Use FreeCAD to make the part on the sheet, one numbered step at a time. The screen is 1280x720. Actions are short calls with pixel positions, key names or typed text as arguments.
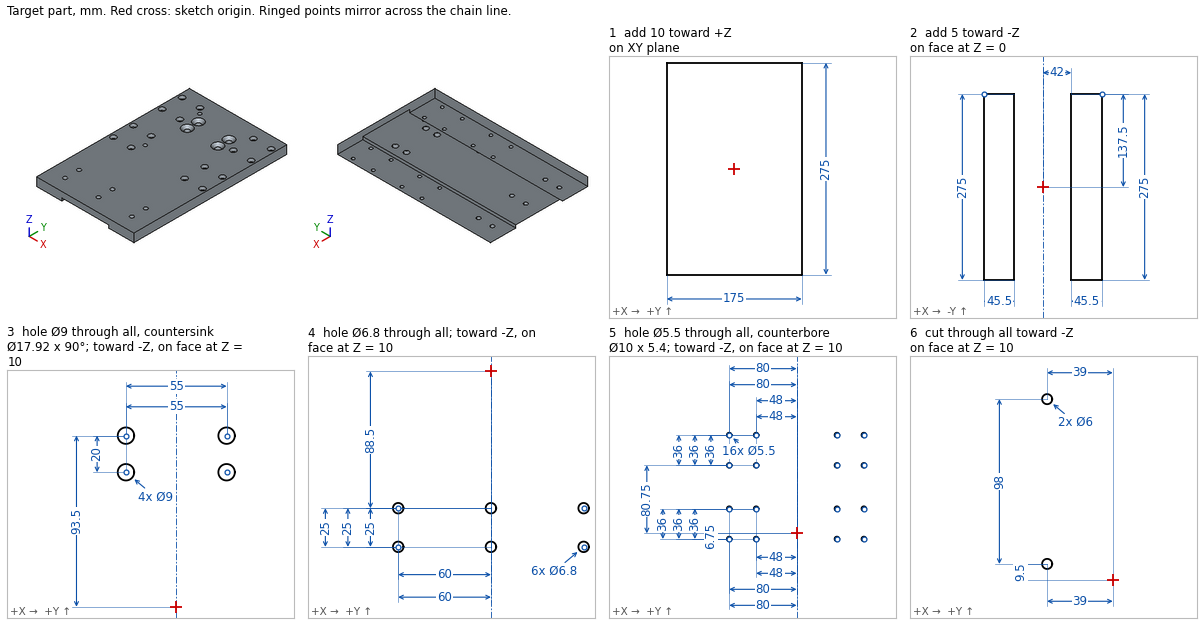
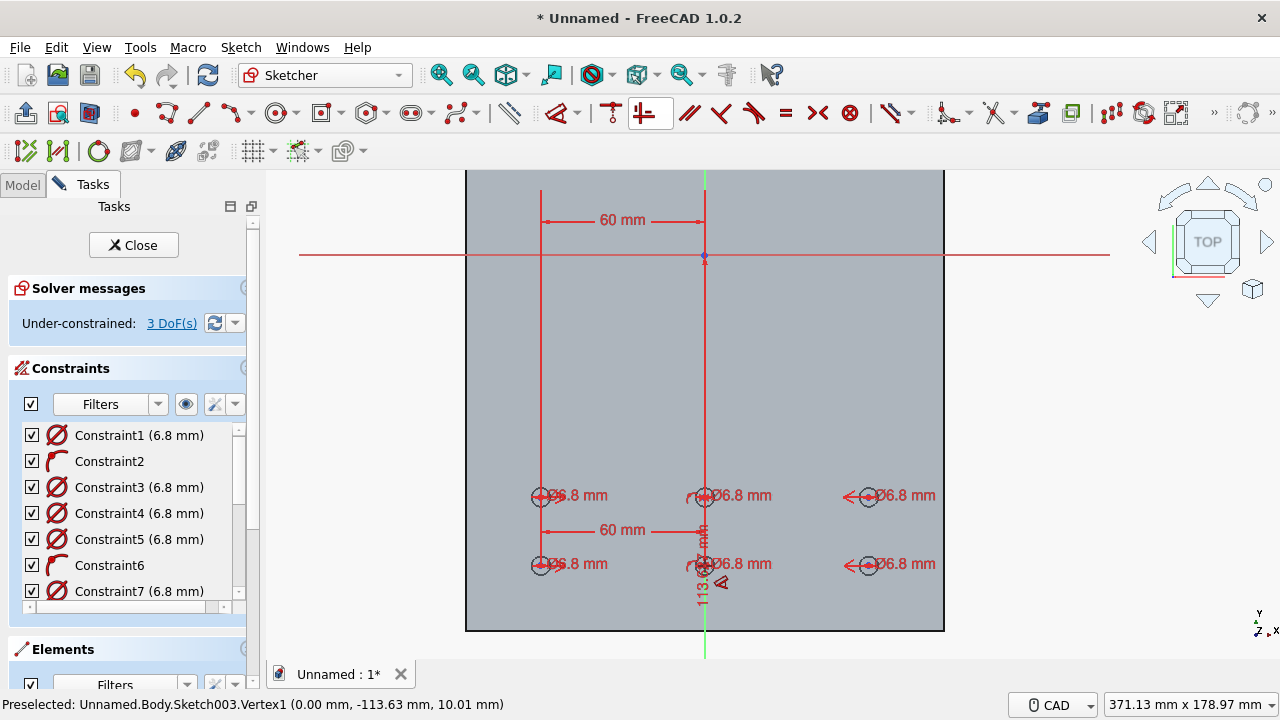
click(705, 497)
click(739, 532)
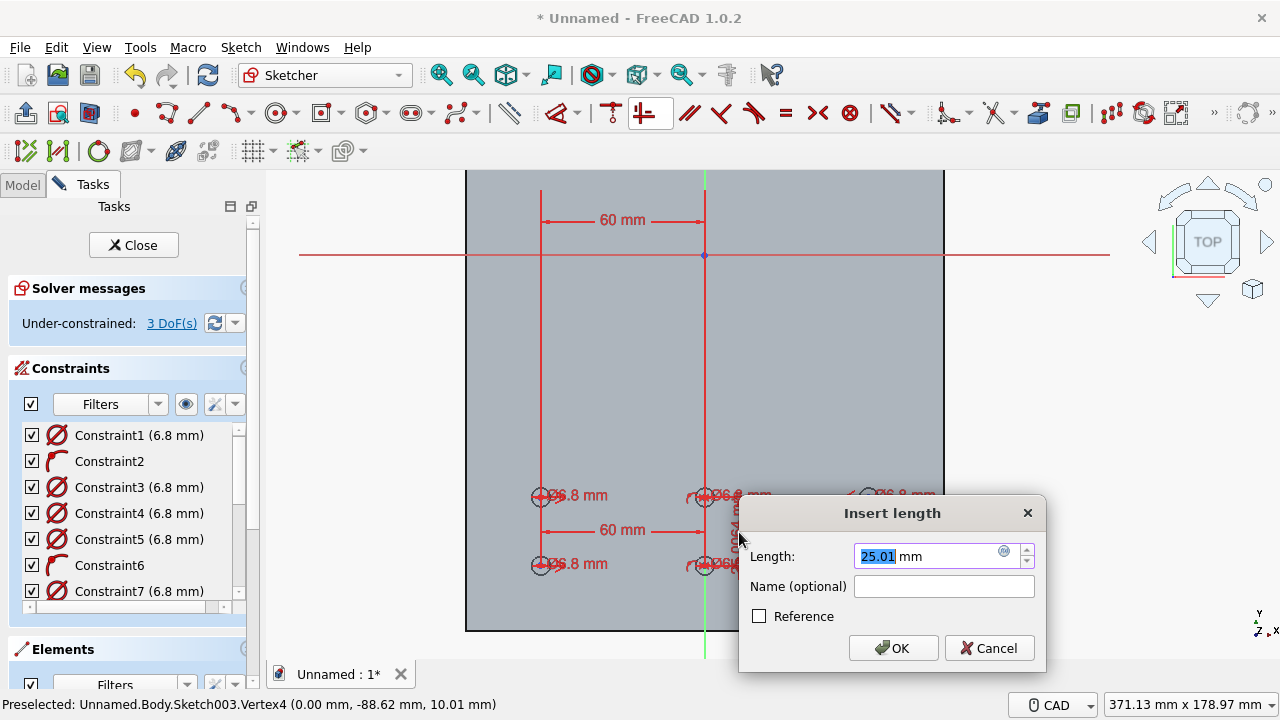
text(25)
key(Return)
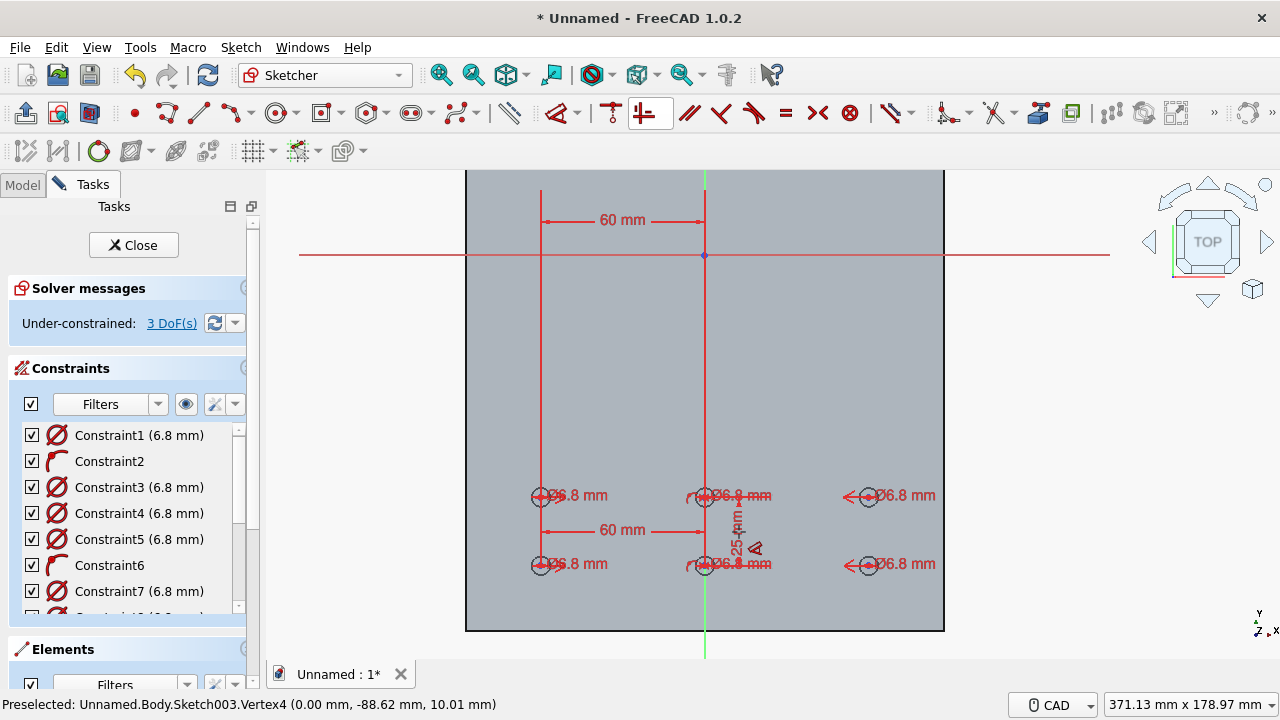
click(541, 566)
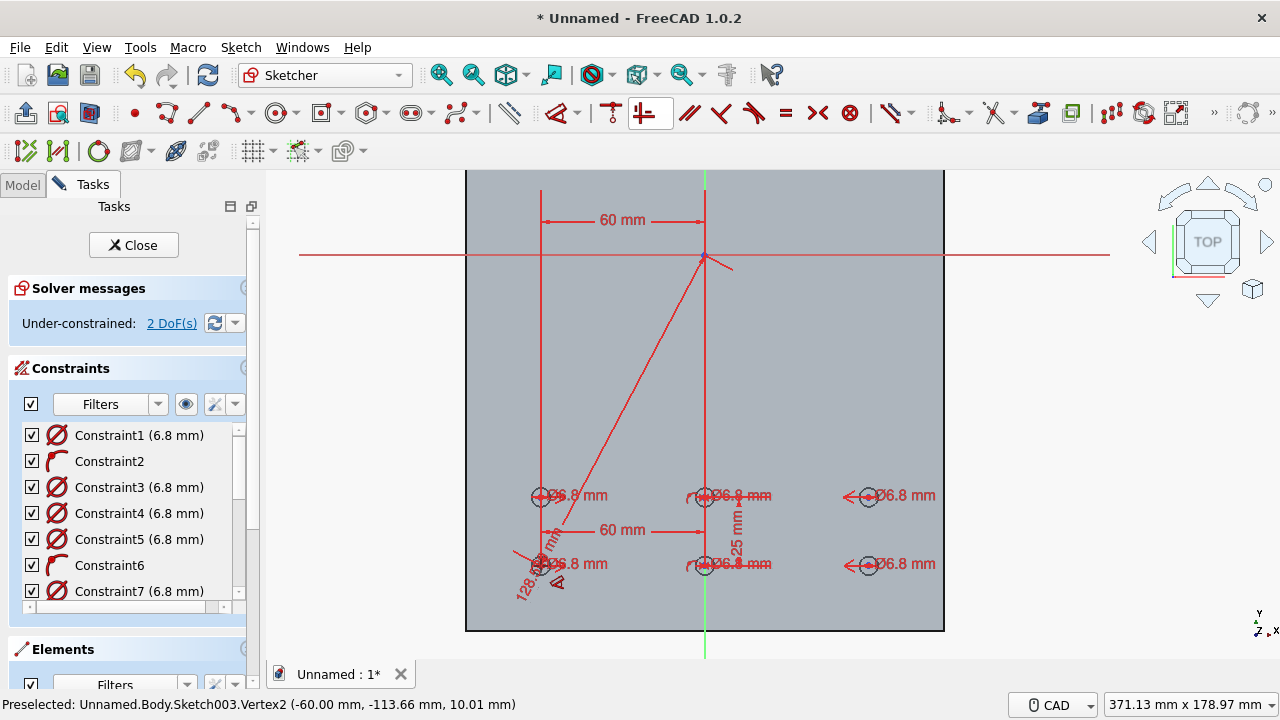
click(705, 497)
click(507, 532)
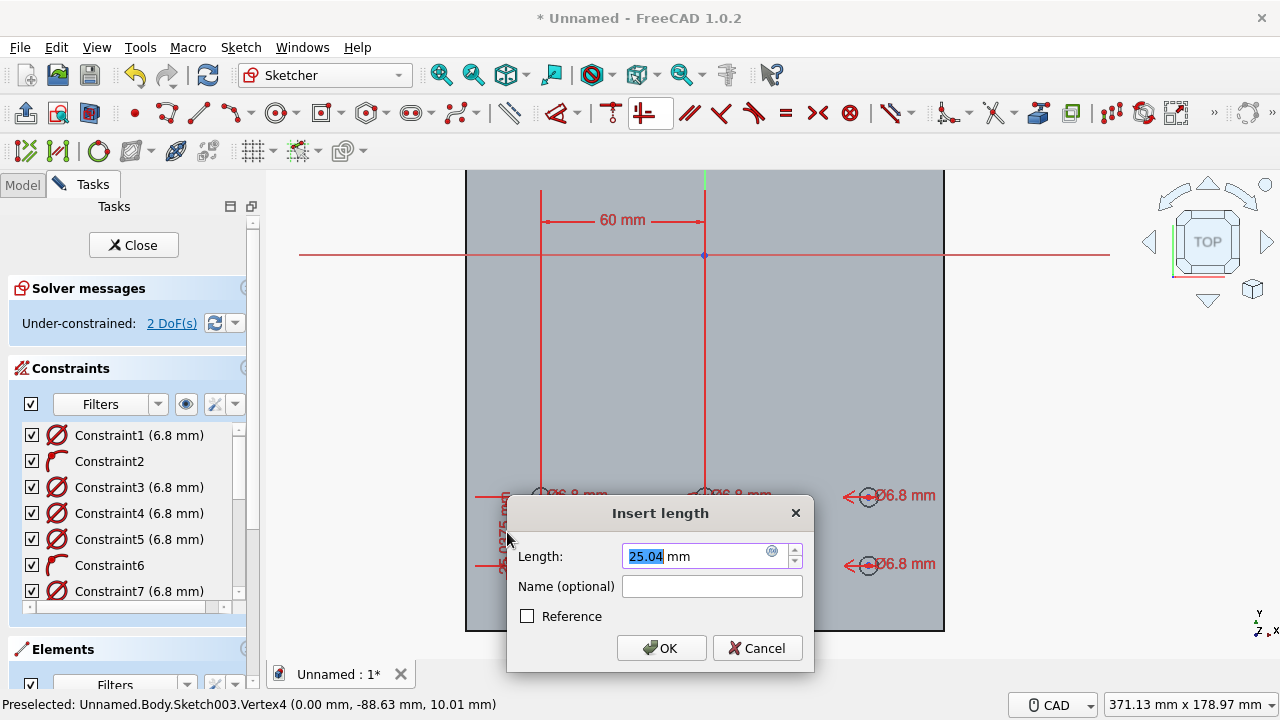
text(25)
key(Return)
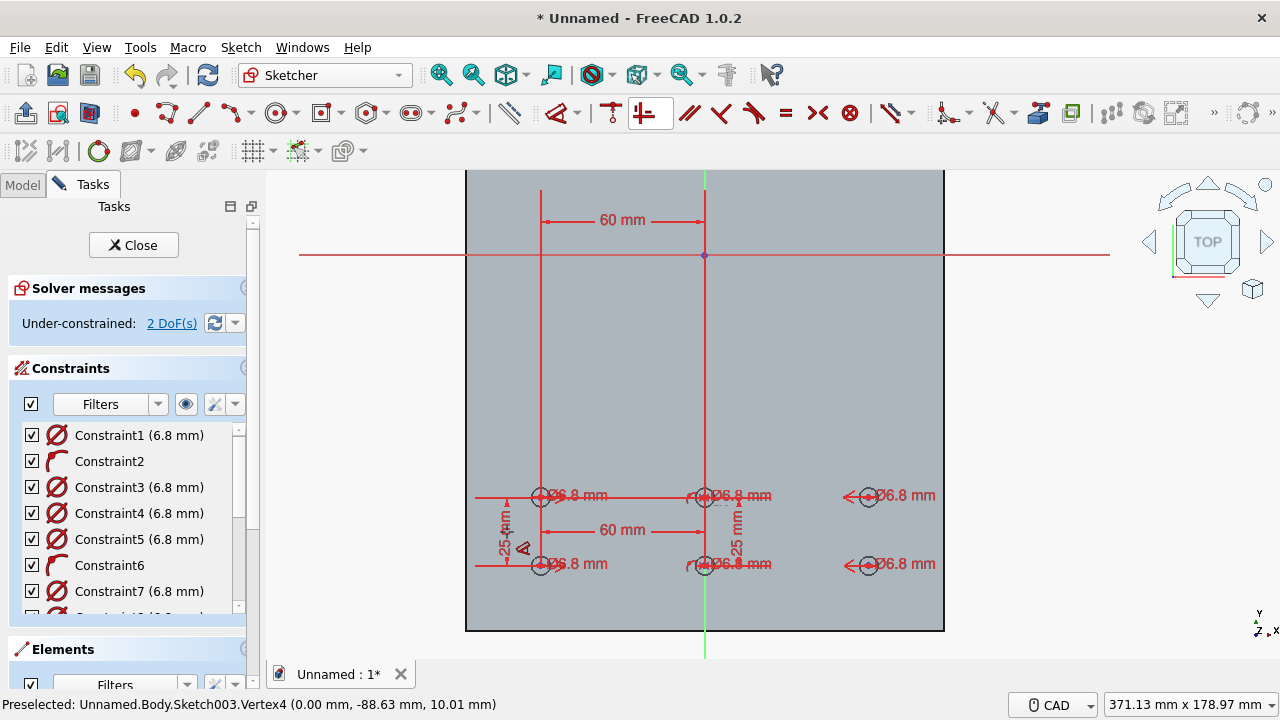
click(541, 566)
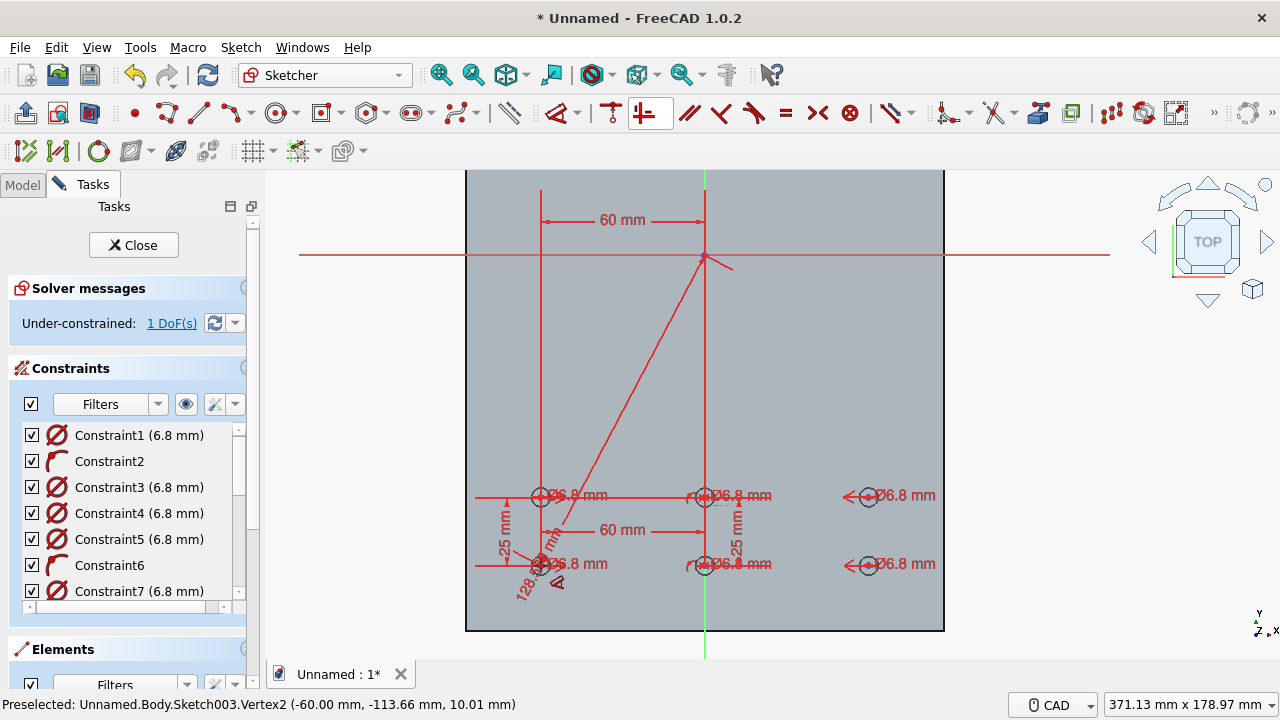
click(541, 497)
click(507, 508)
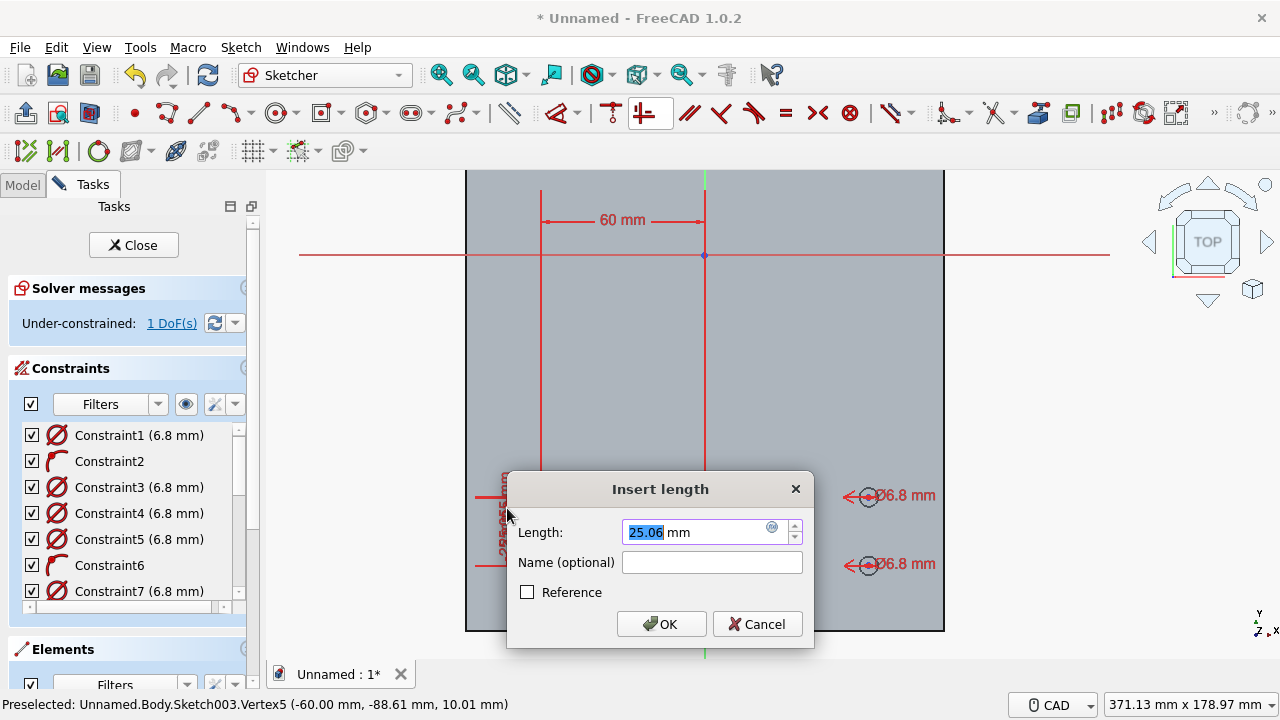
text(25)
key(Return)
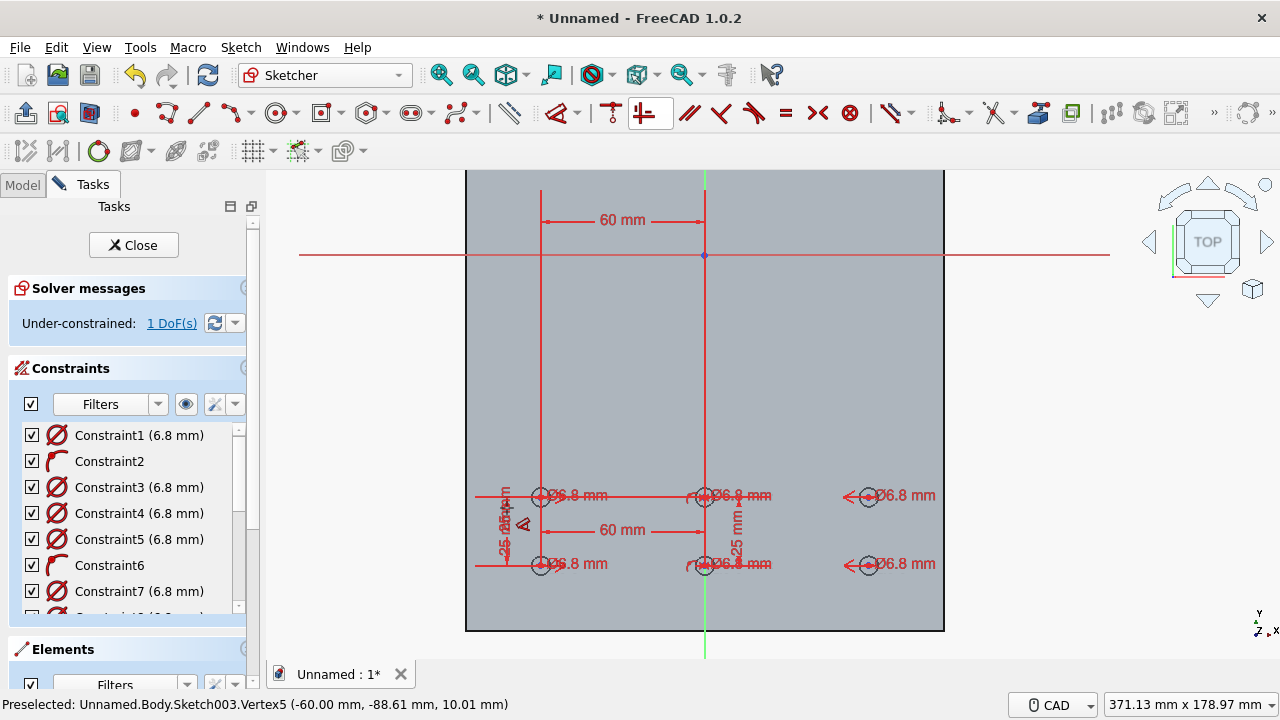
click(705, 497)
click(739, 376)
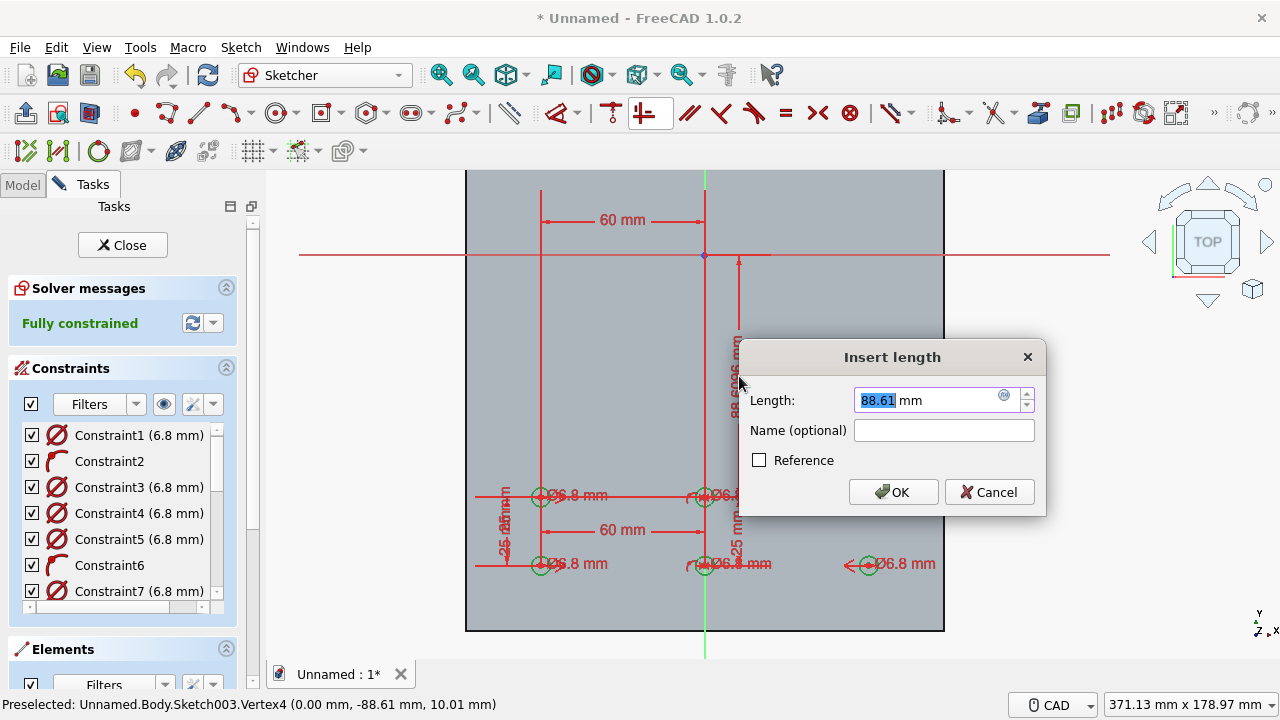
text(88.5)
key(Return)
key(Escape)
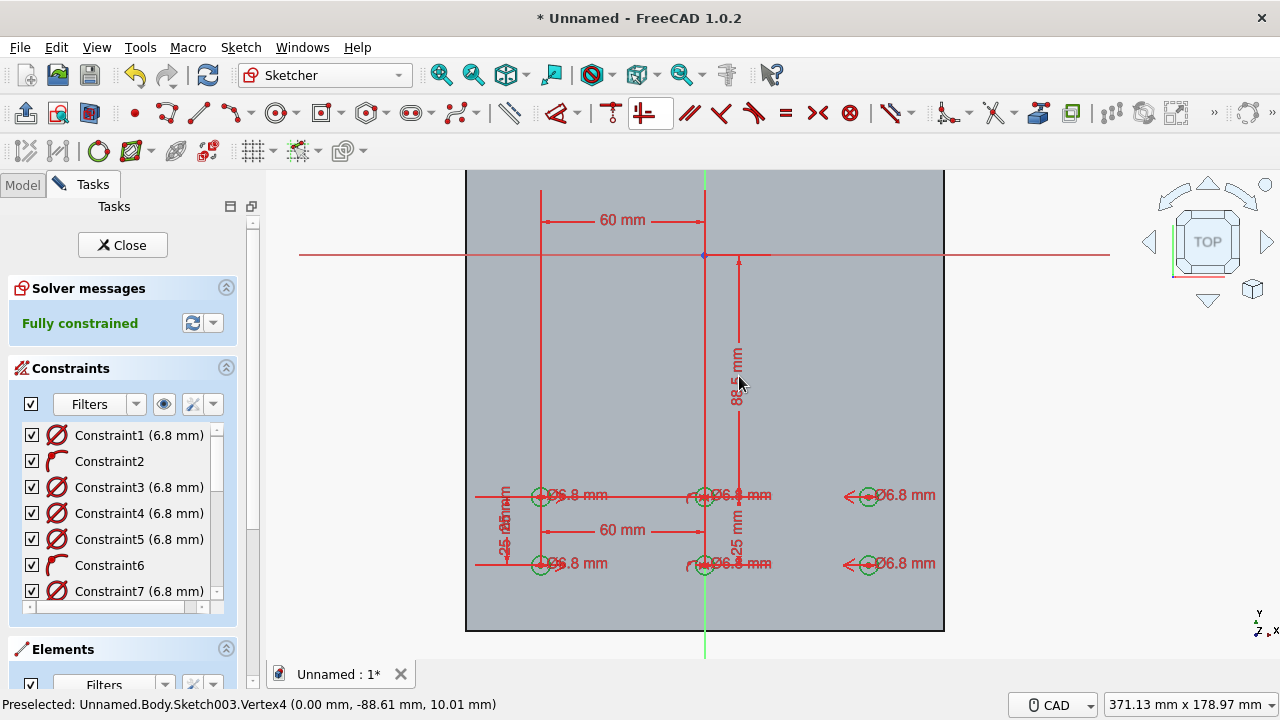
click(123, 245)